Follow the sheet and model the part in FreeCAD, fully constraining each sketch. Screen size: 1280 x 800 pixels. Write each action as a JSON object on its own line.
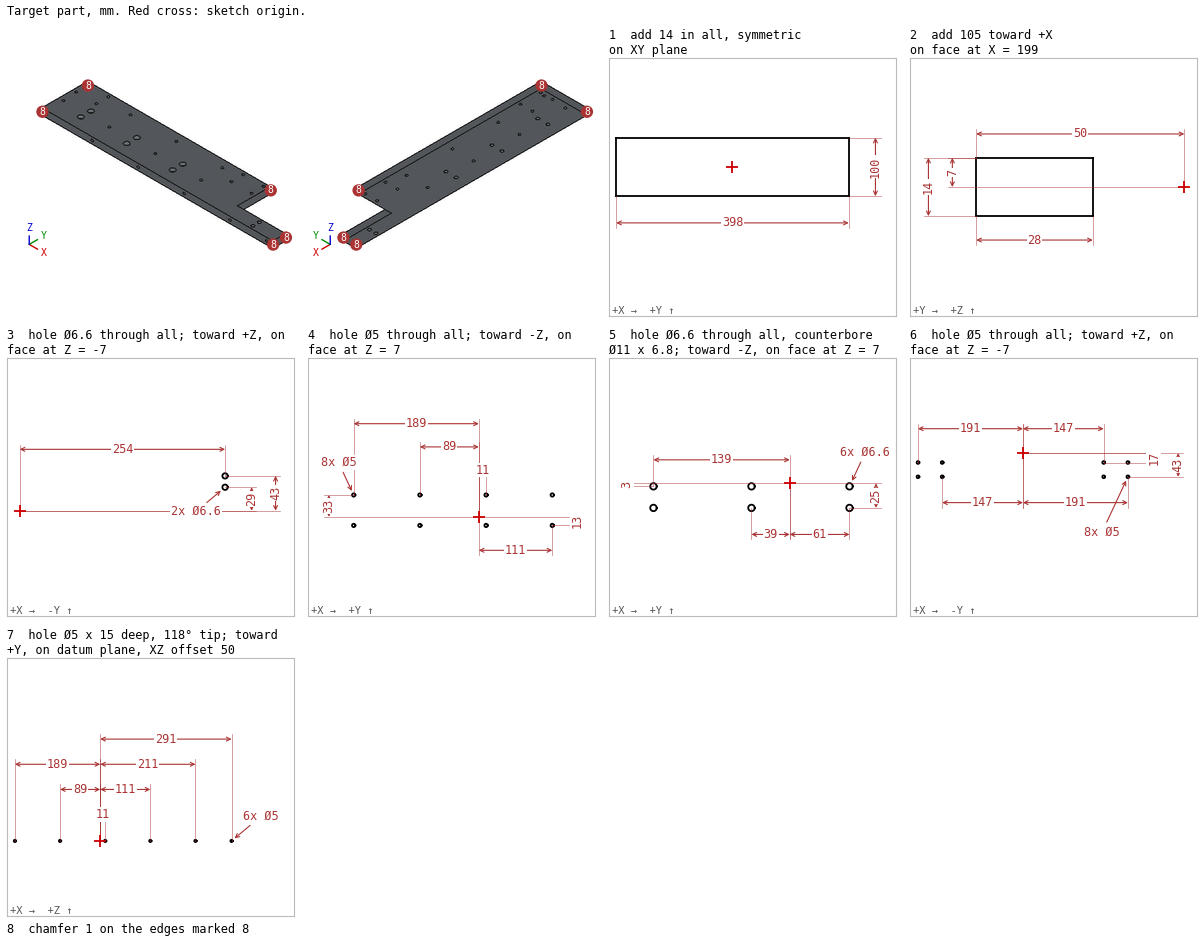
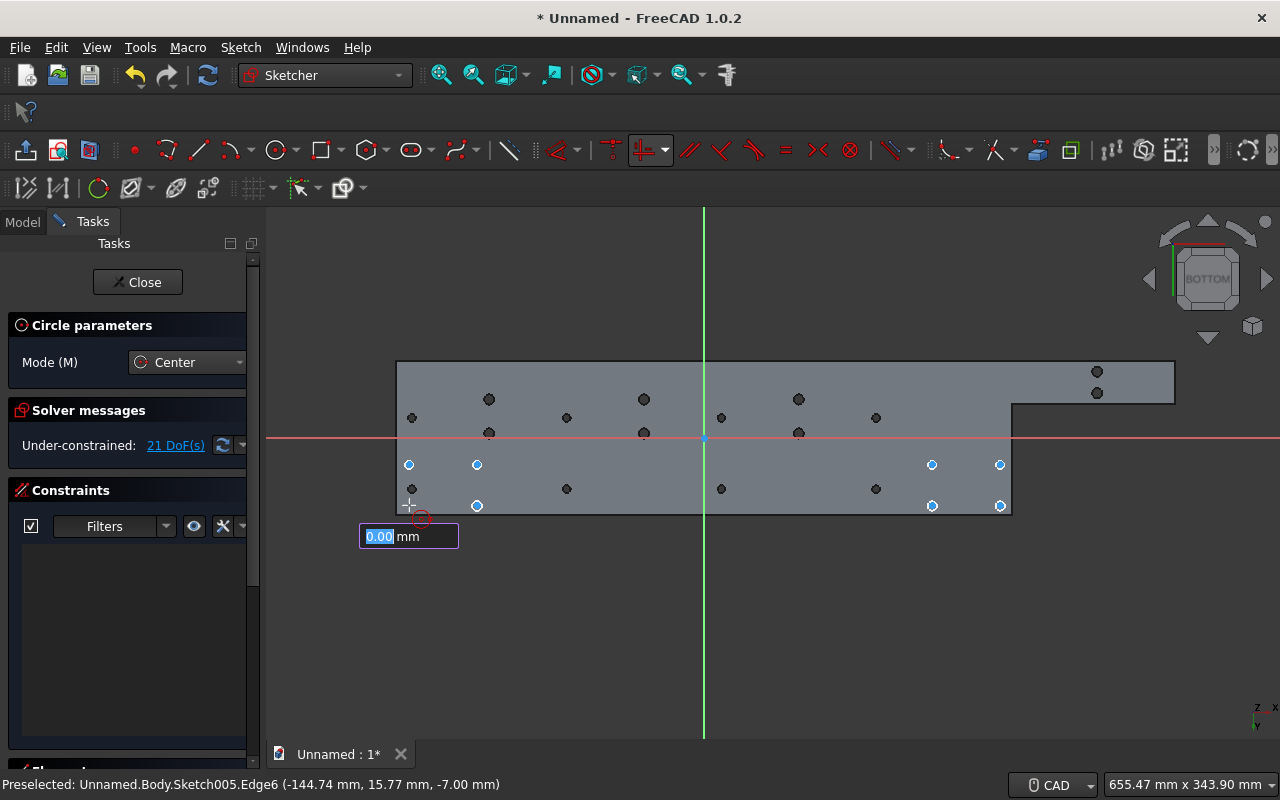
{"action": "scroll", "coordinate": [412, 502], "scroll_direction": "up", "scroll_amount": 8}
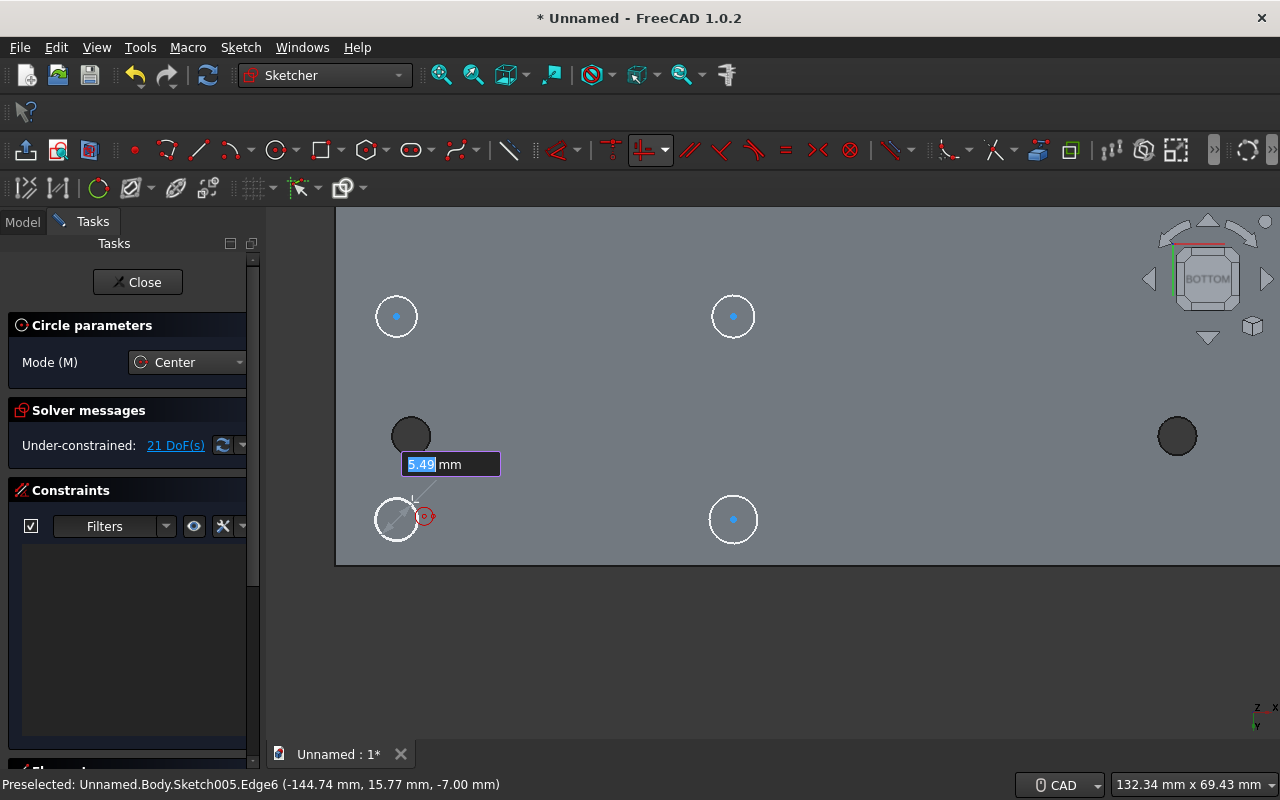
{"action": "left_click", "coordinate": [409, 499]}
{"action": "key", "text": "Escape"}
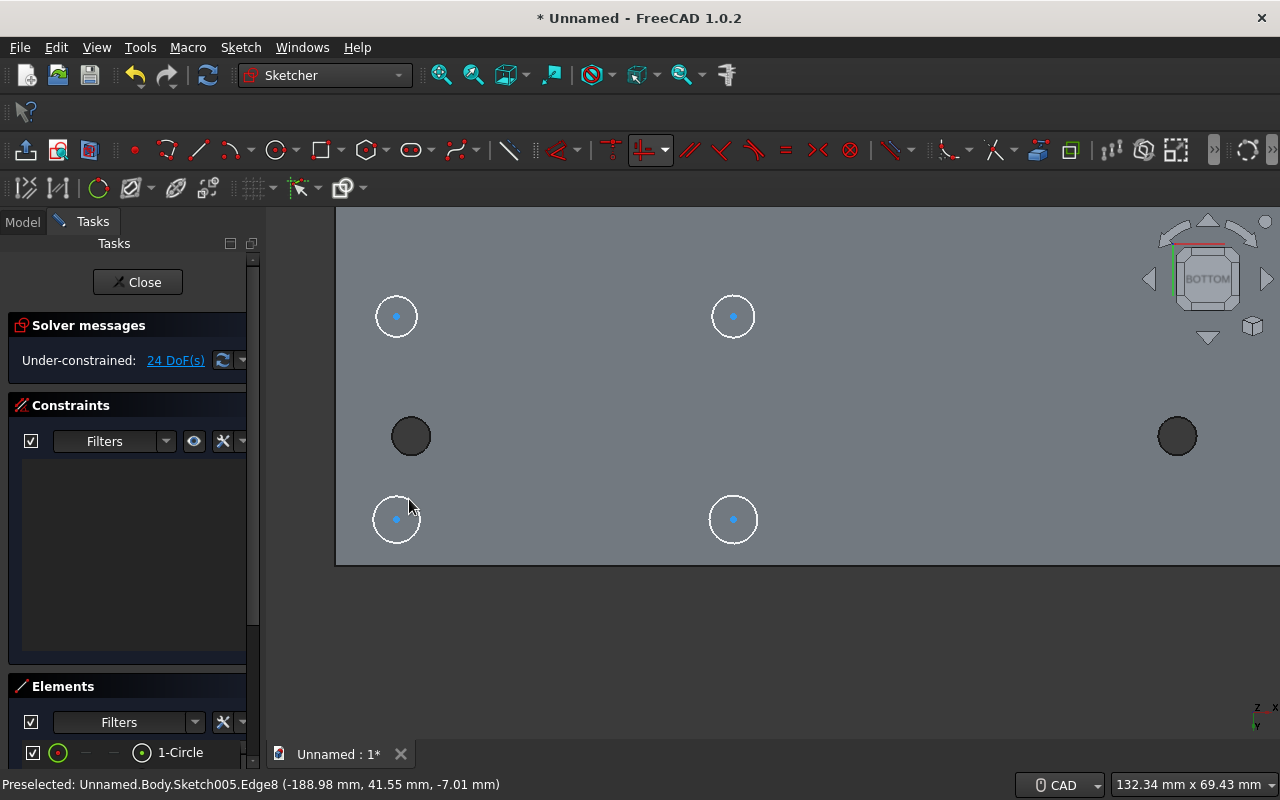
{"action": "scroll", "coordinate": [412, 502], "scroll_direction": "down", "scroll_amount": 8}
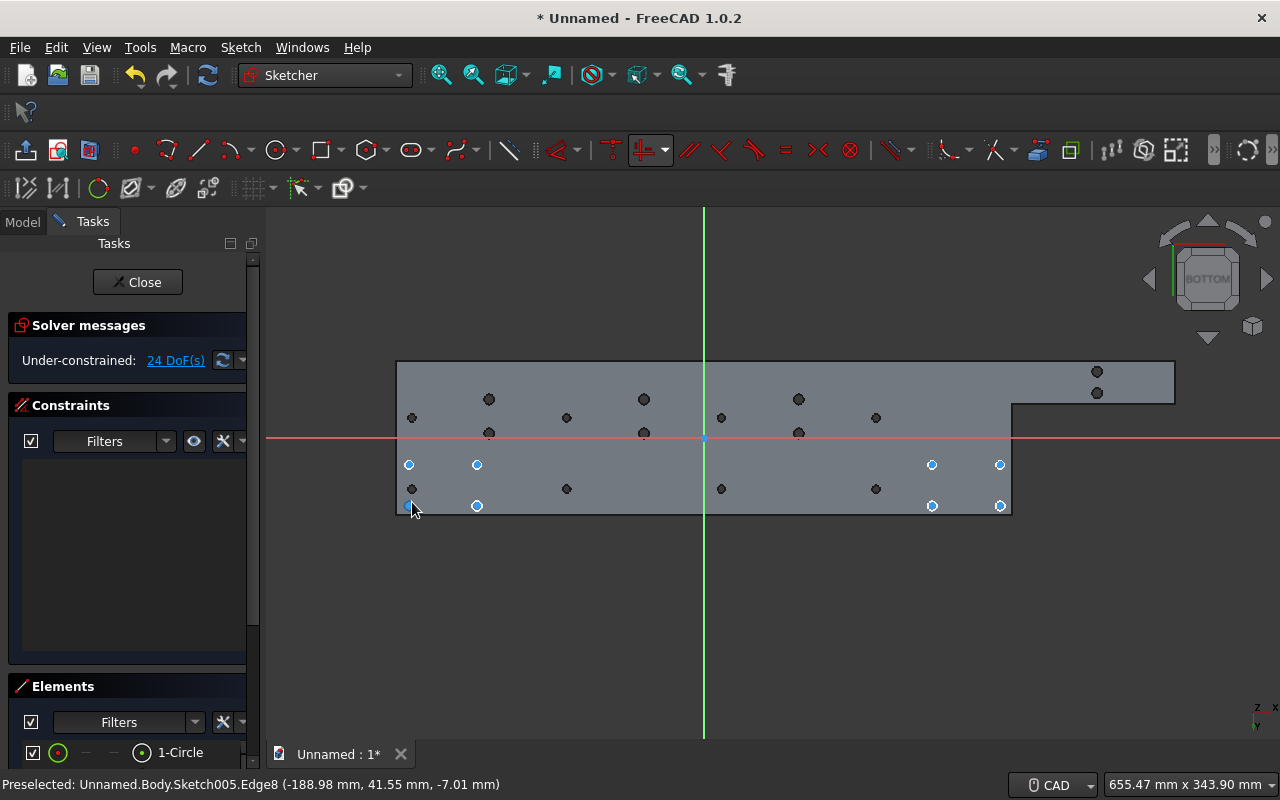
{"action": "scroll", "coordinate": [1003, 503], "scroll_direction": "up", "scroll_amount": 6}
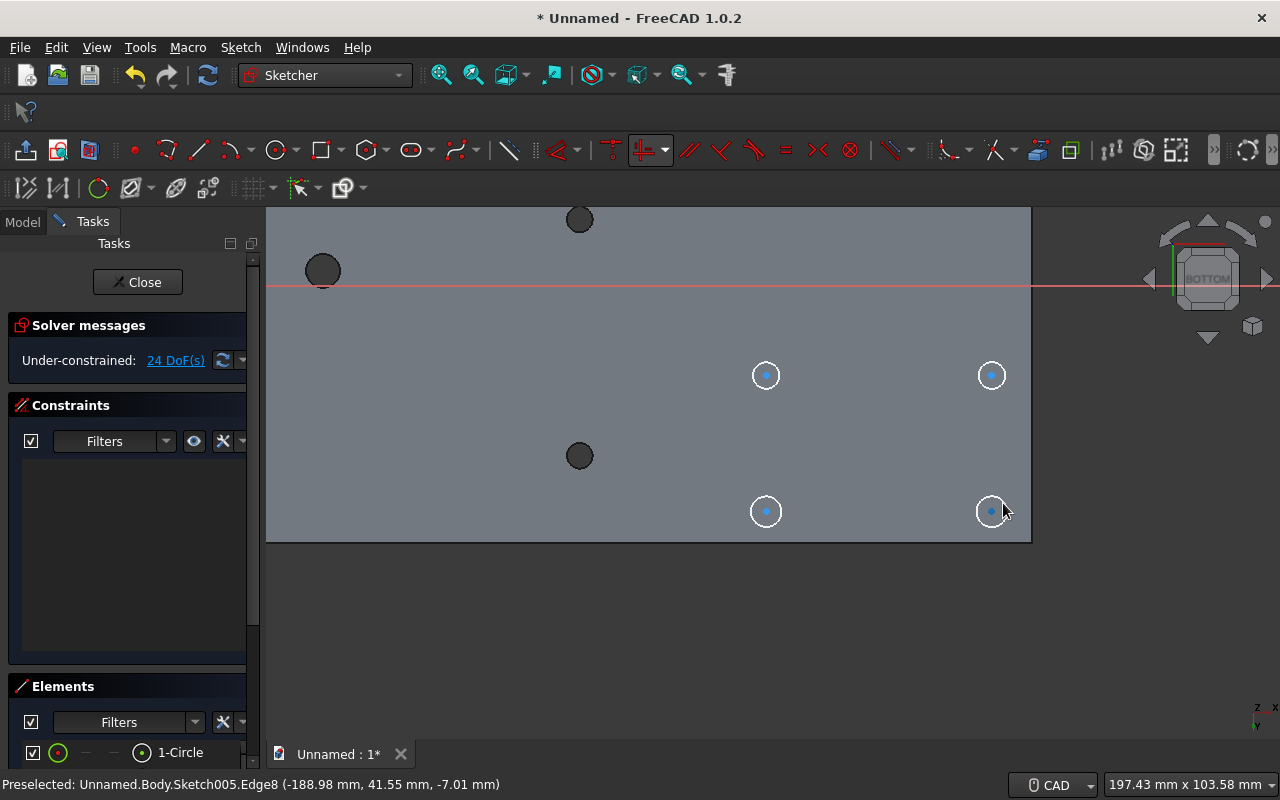
{"action": "left_click", "coordinate": [1003, 501]}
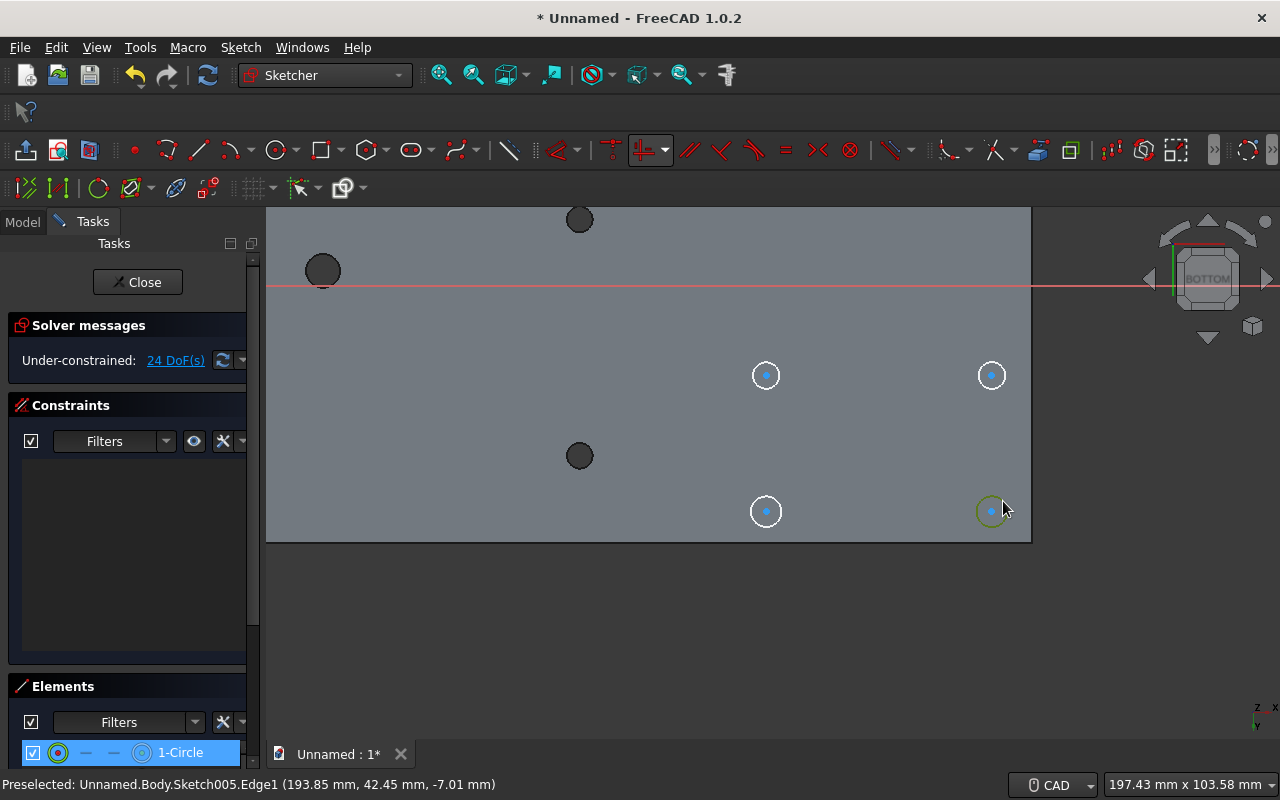
{"action": "left_click", "coordinate": [775, 366]}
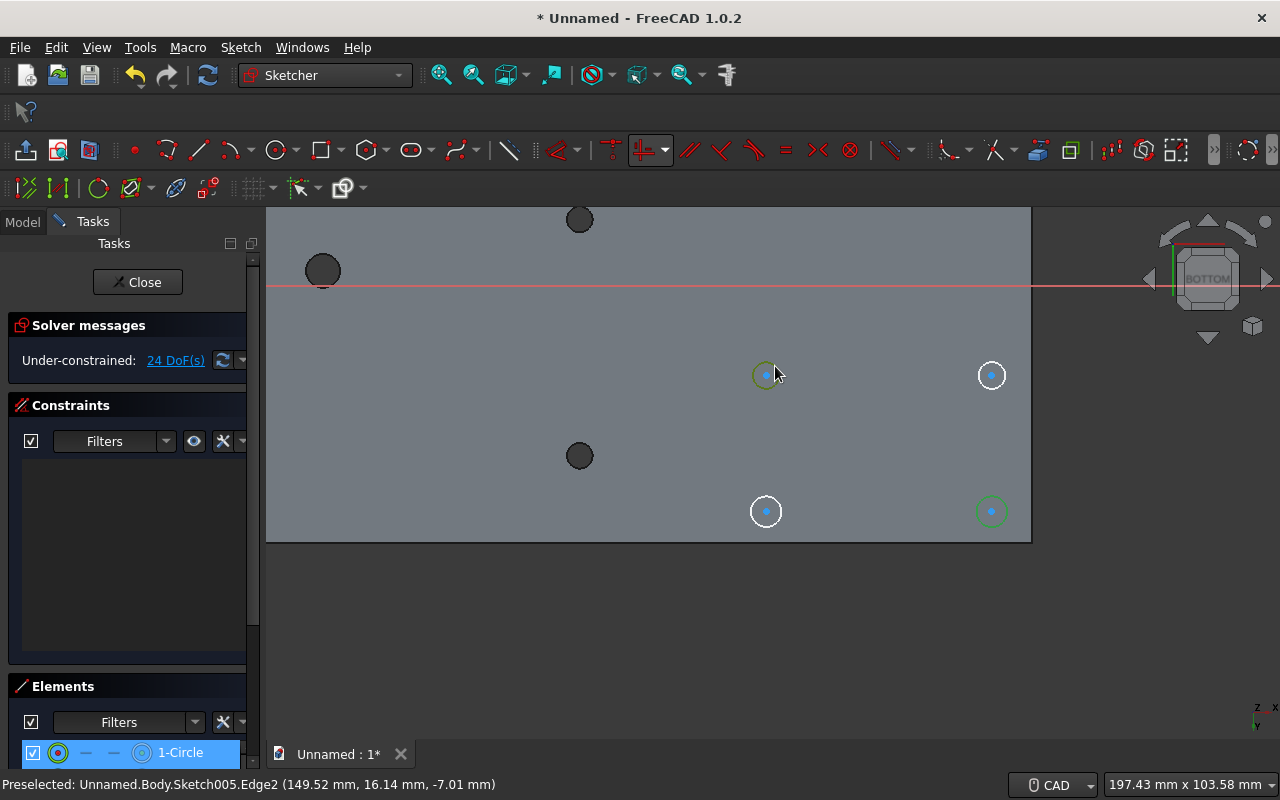
{"action": "left_click", "coordinate": [1001, 366]}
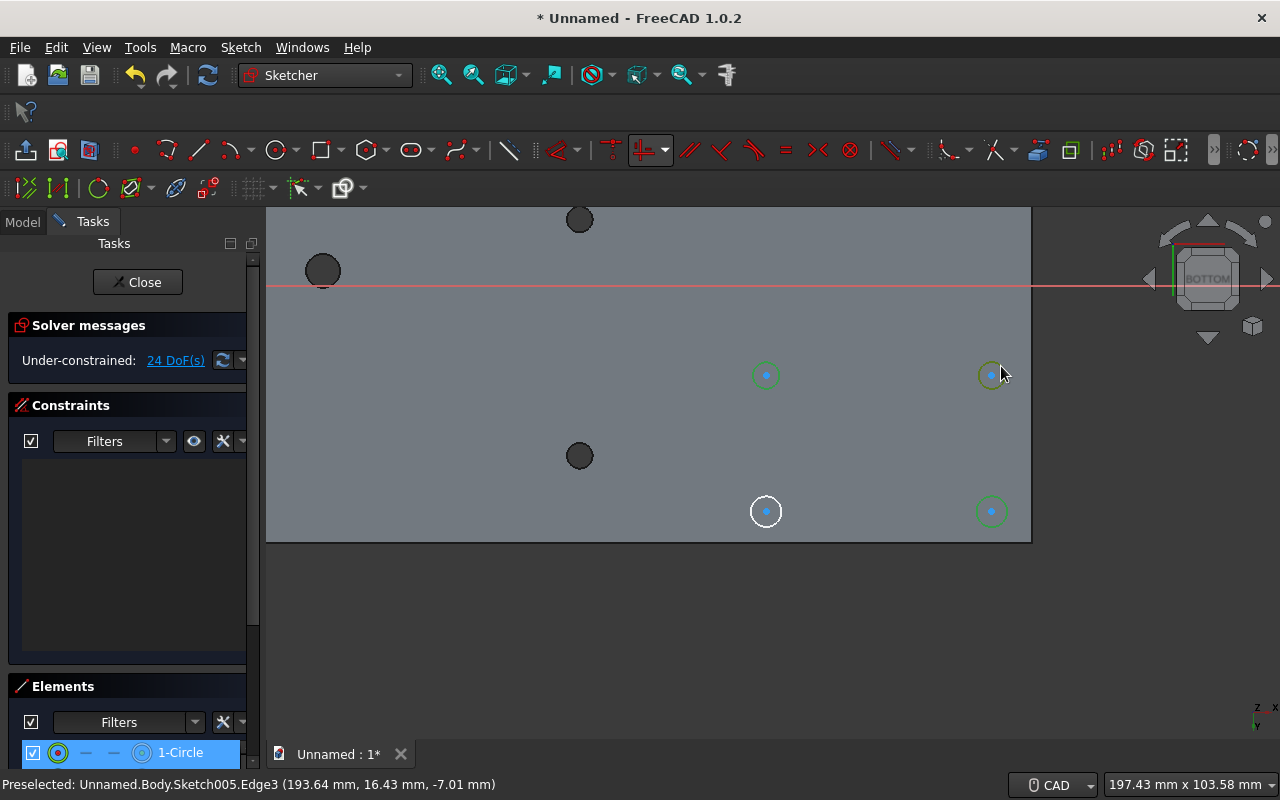
{"action": "left_click", "coordinate": [777, 501]}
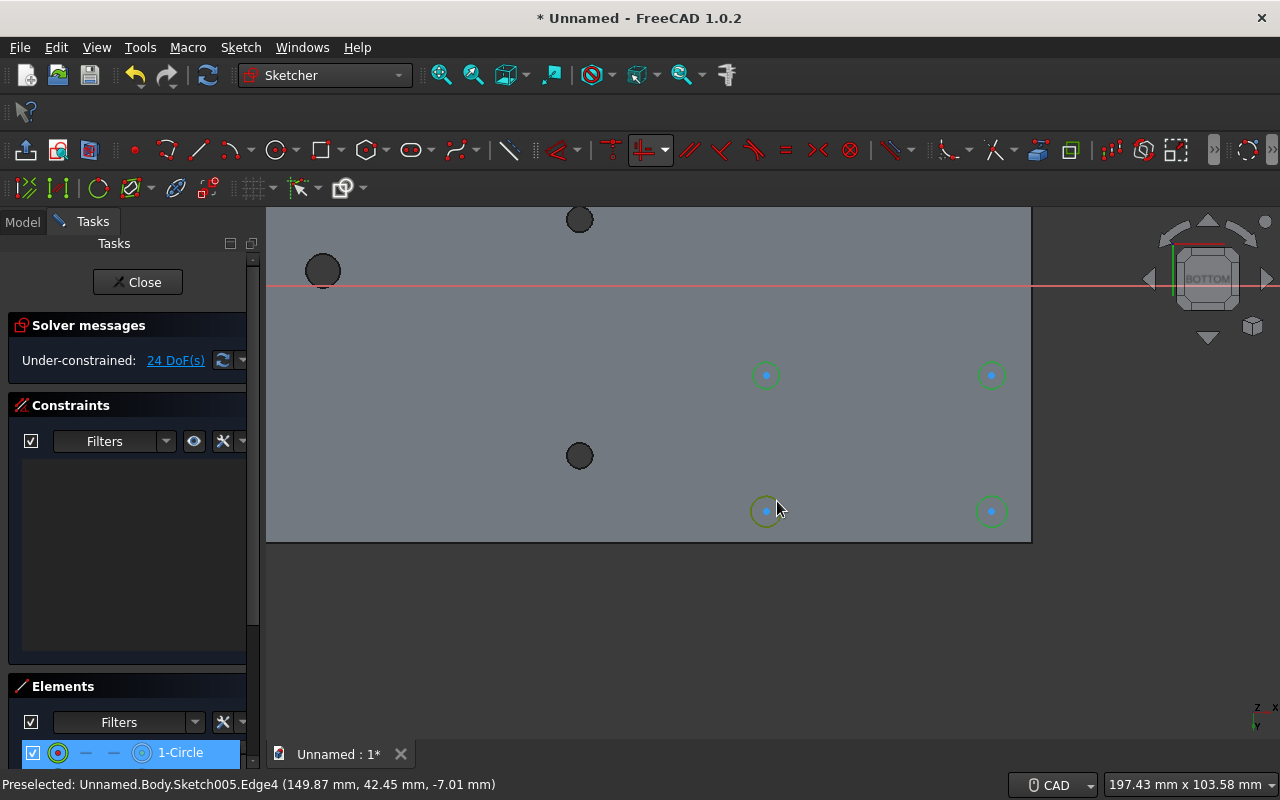
{"action": "scroll", "coordinate": [1004, 503], "scroll_direction": "down", "scroll_amount": 6}